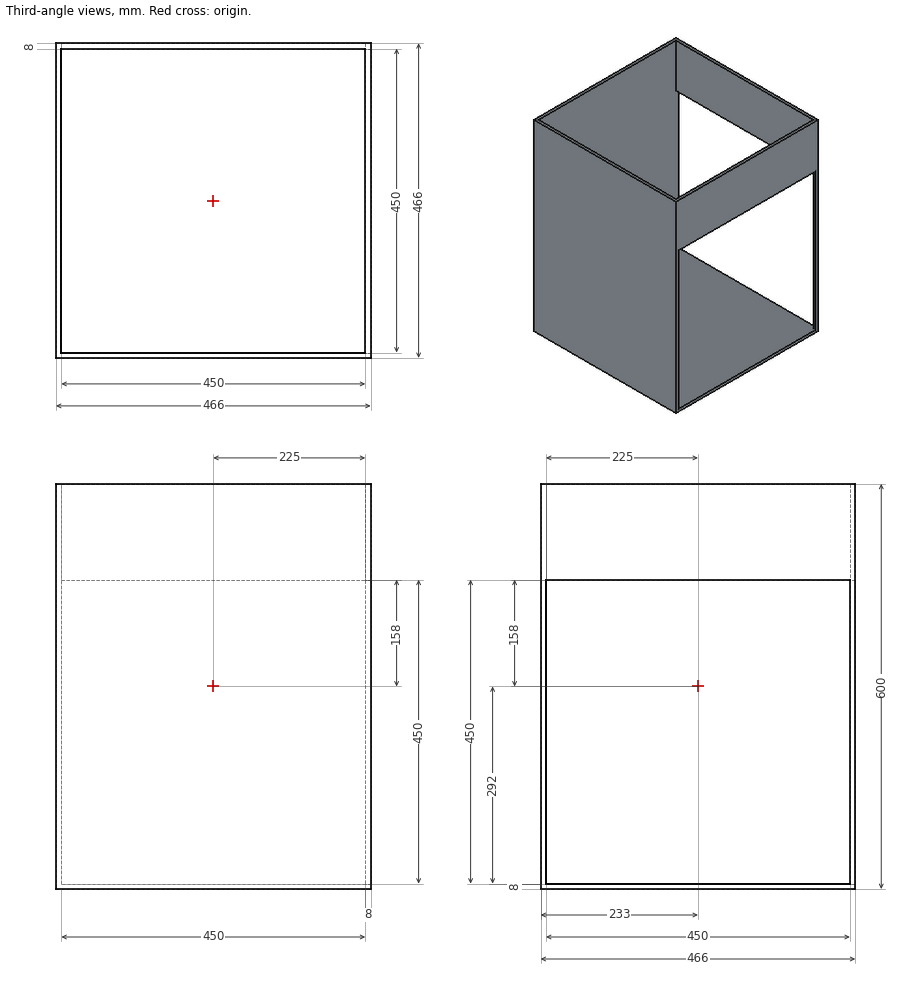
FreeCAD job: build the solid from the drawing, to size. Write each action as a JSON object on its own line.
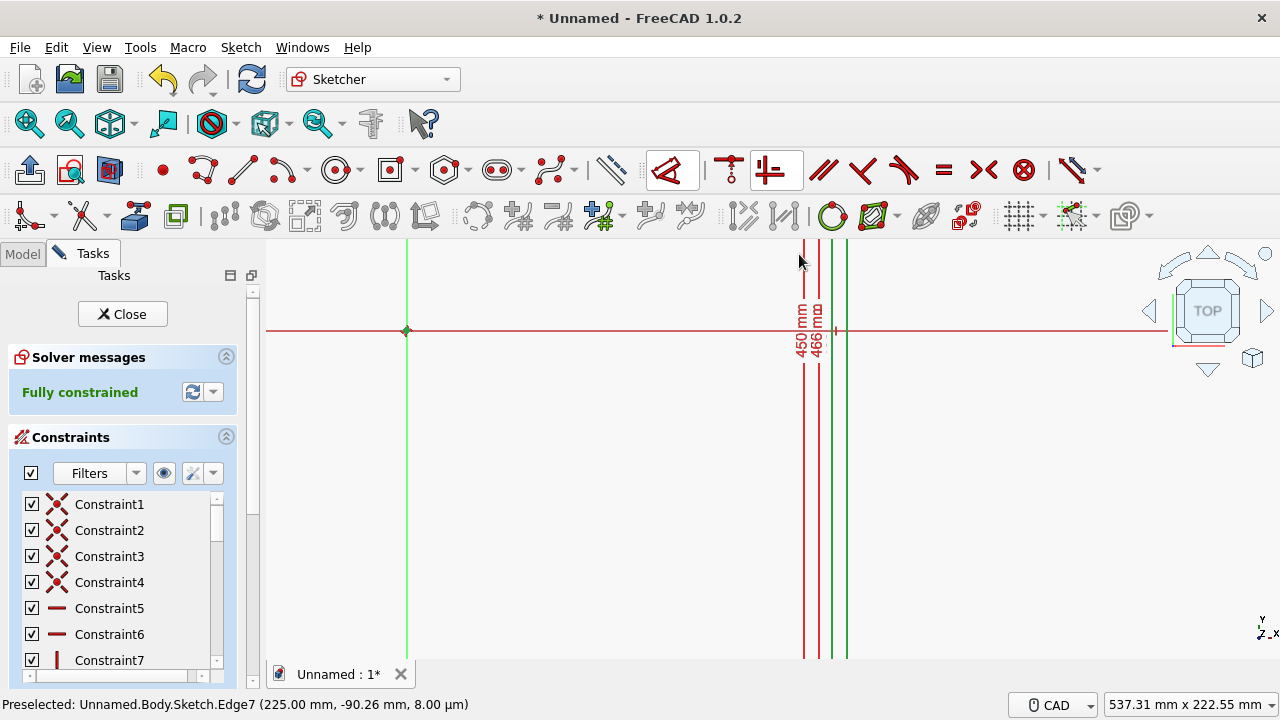
{"action": "left_click", "coordinate": [123, 314]}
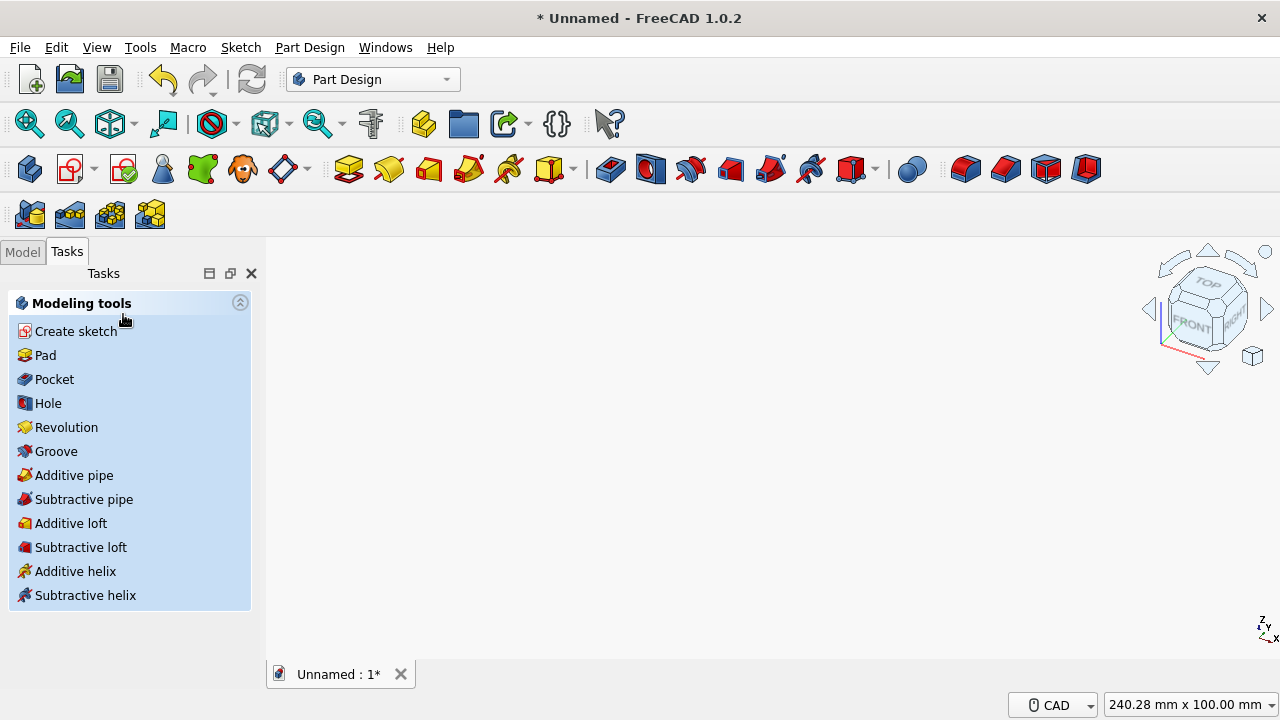
{"action": "left_click", "coordinate": [350, 170]}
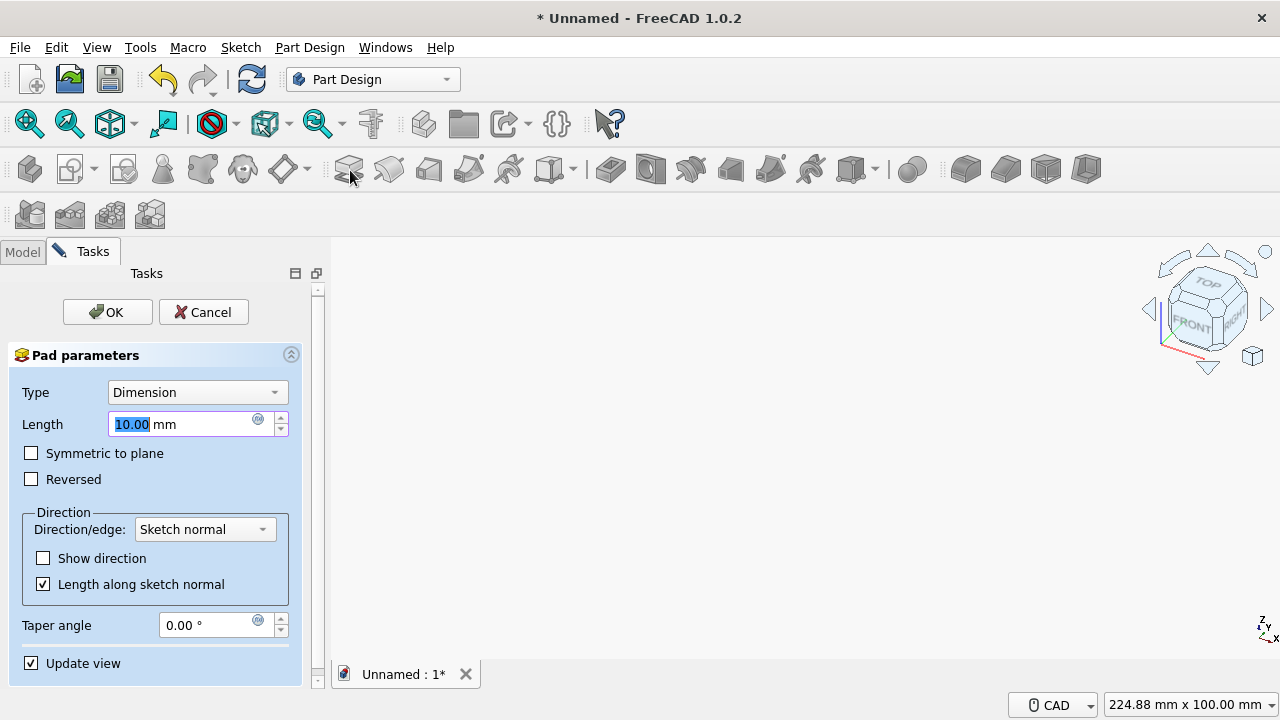
{"action": "type", "text": "600"}
{"action": "key", "text": "Tab"}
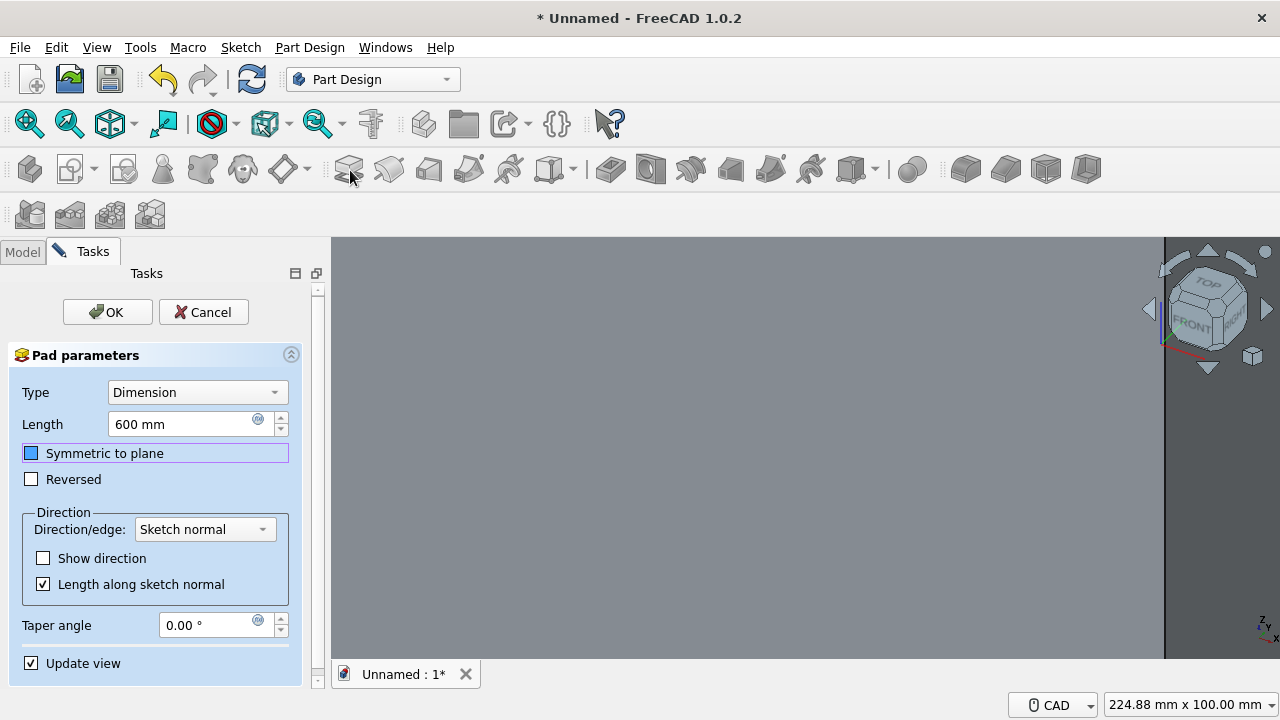
{"action": "left_click", "coordinate": [30, 453]}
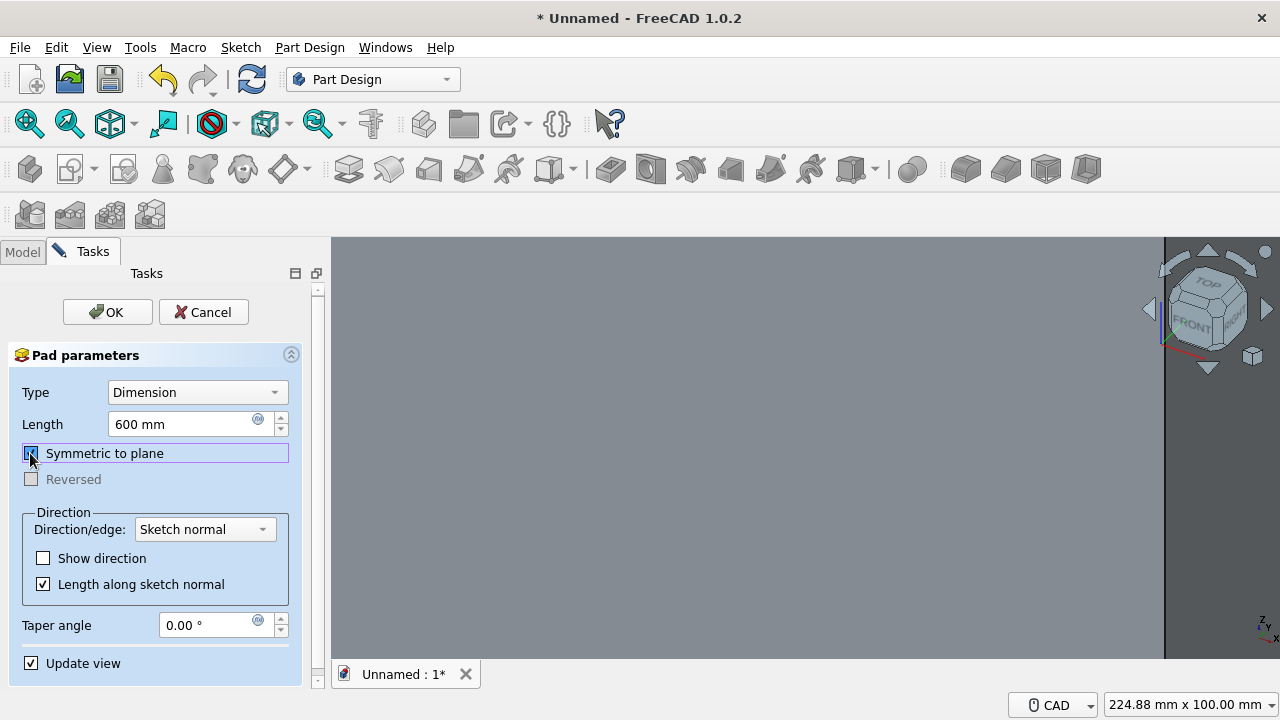
{"action": "left_click", "coordinate": [108, 312]}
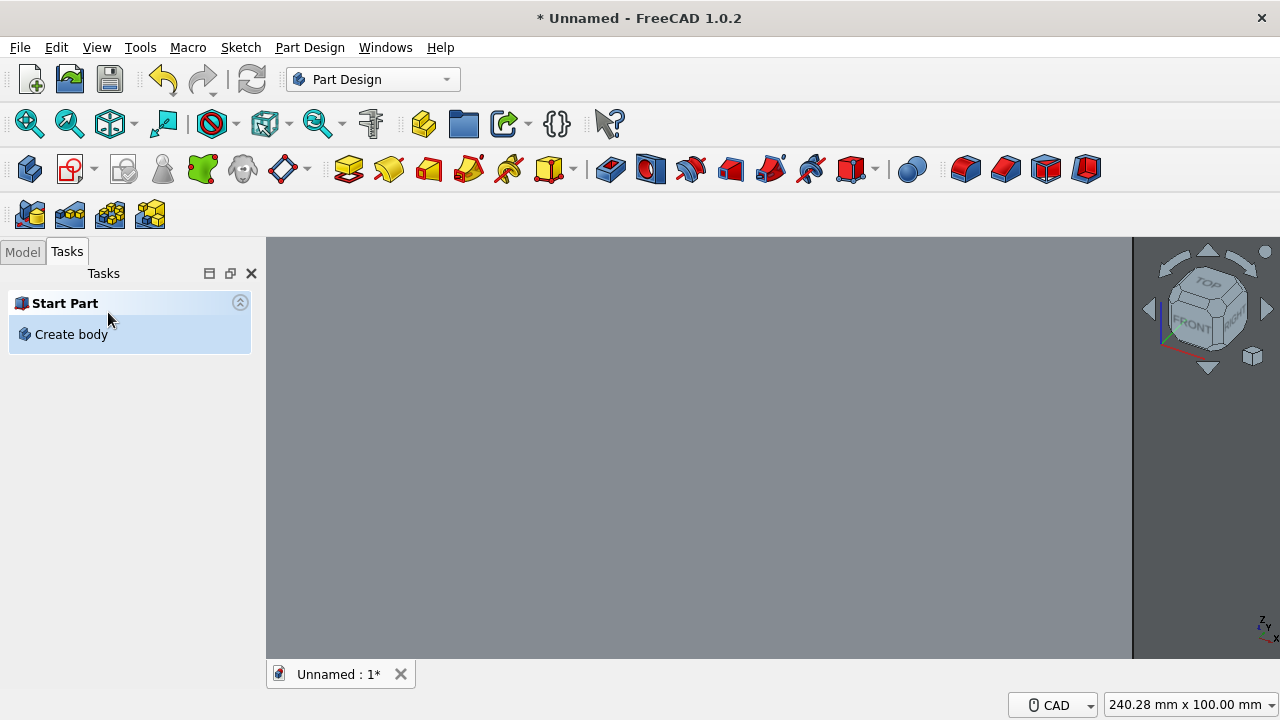
{"action": "left_click", "coordinate": [30, 124]}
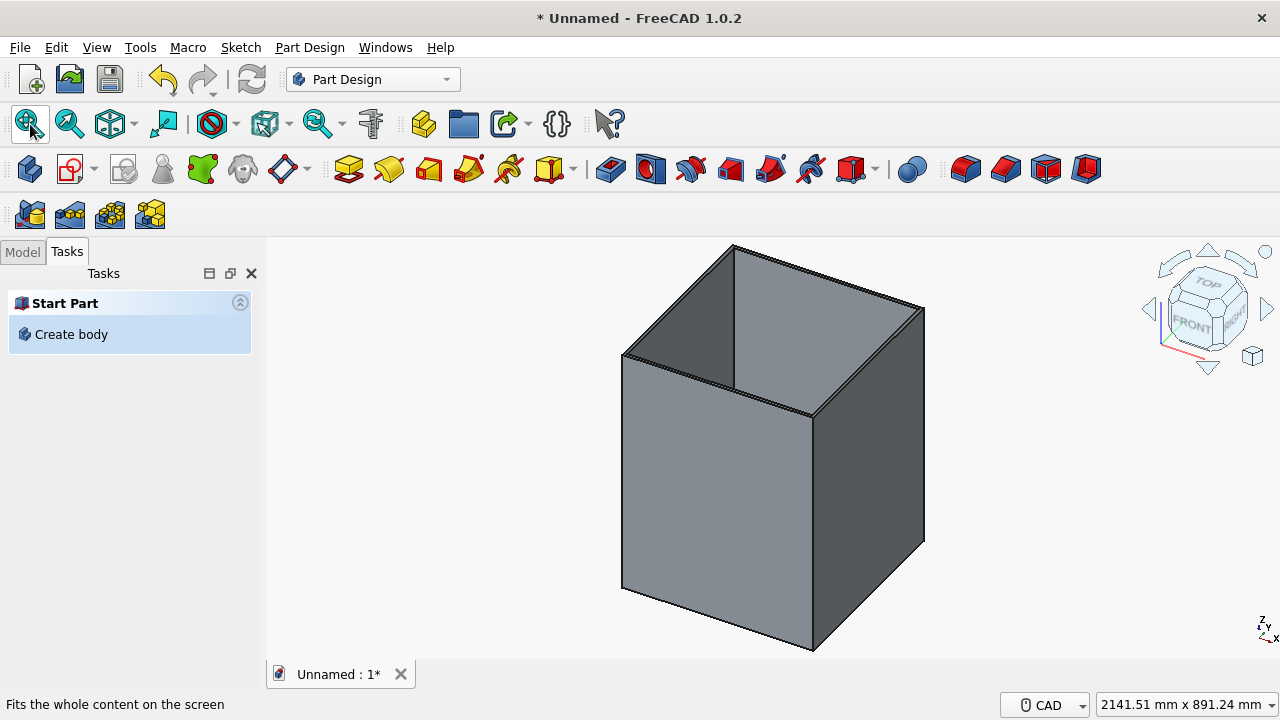
{"action": "left_click", "coordinate": [23, 251]}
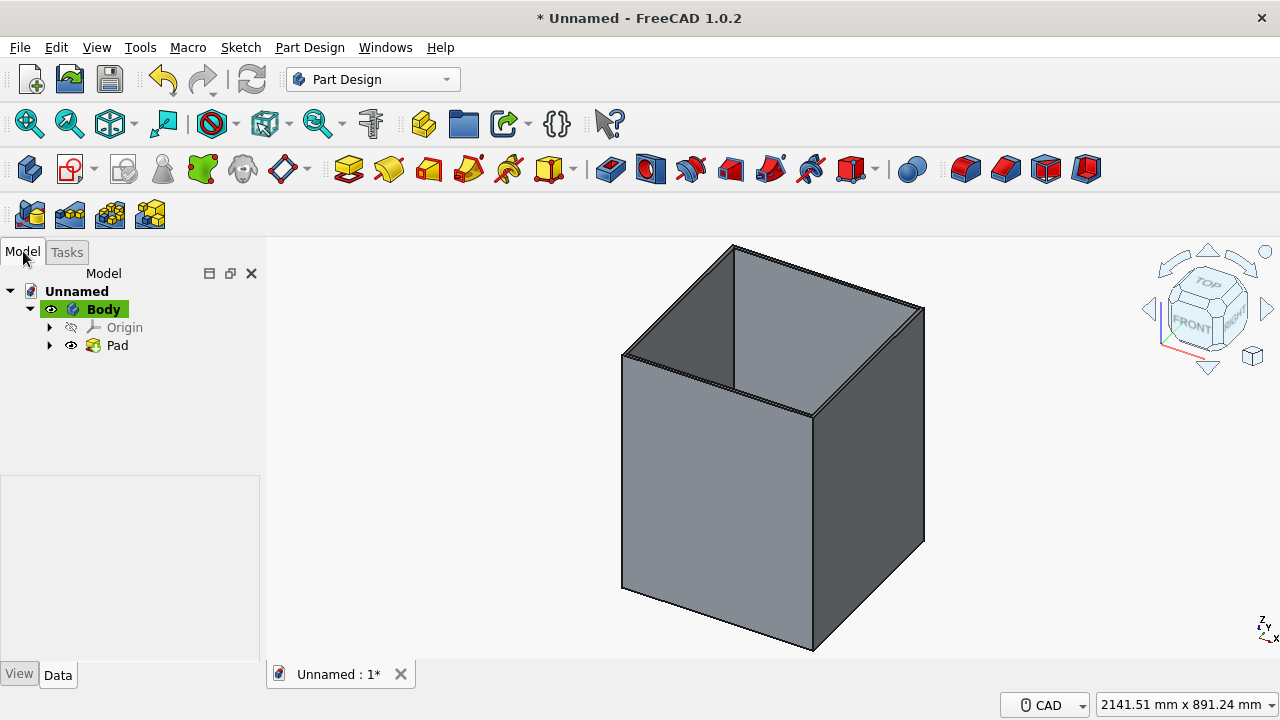
{"action": "left_click", "coordinate": [50, 327]}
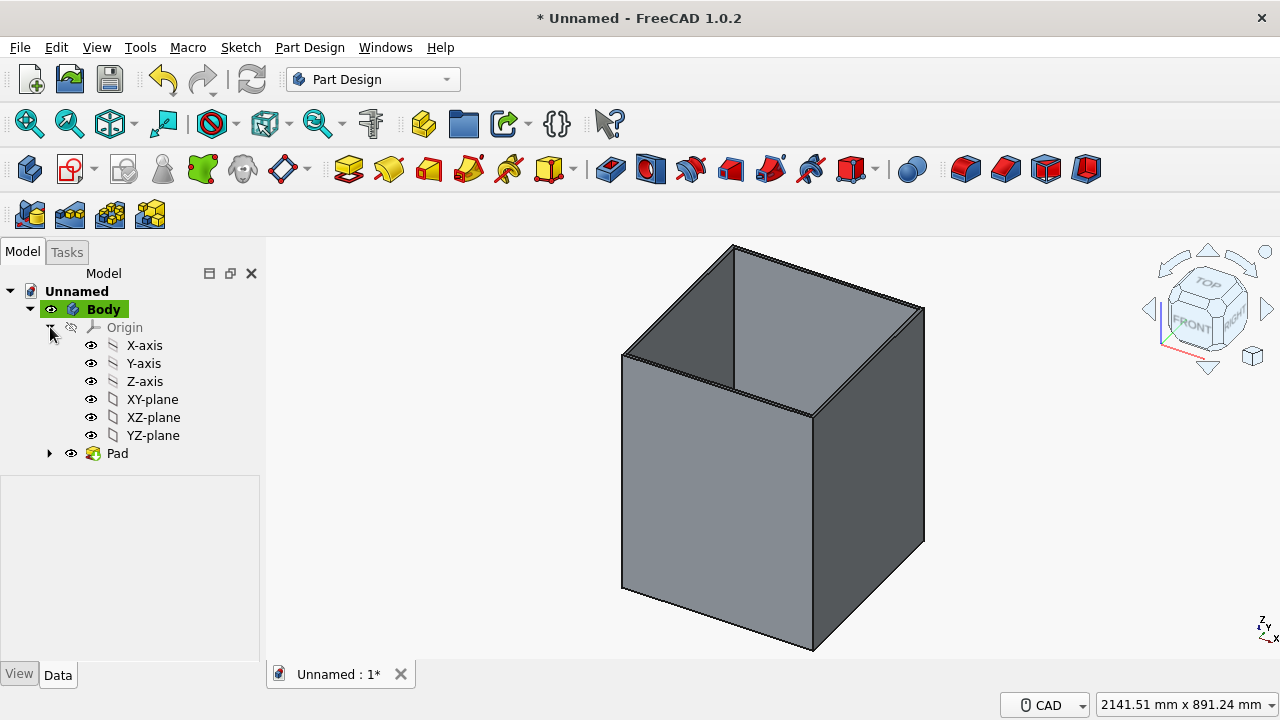
{"action": "left_click", "coordinate": [136, 435]}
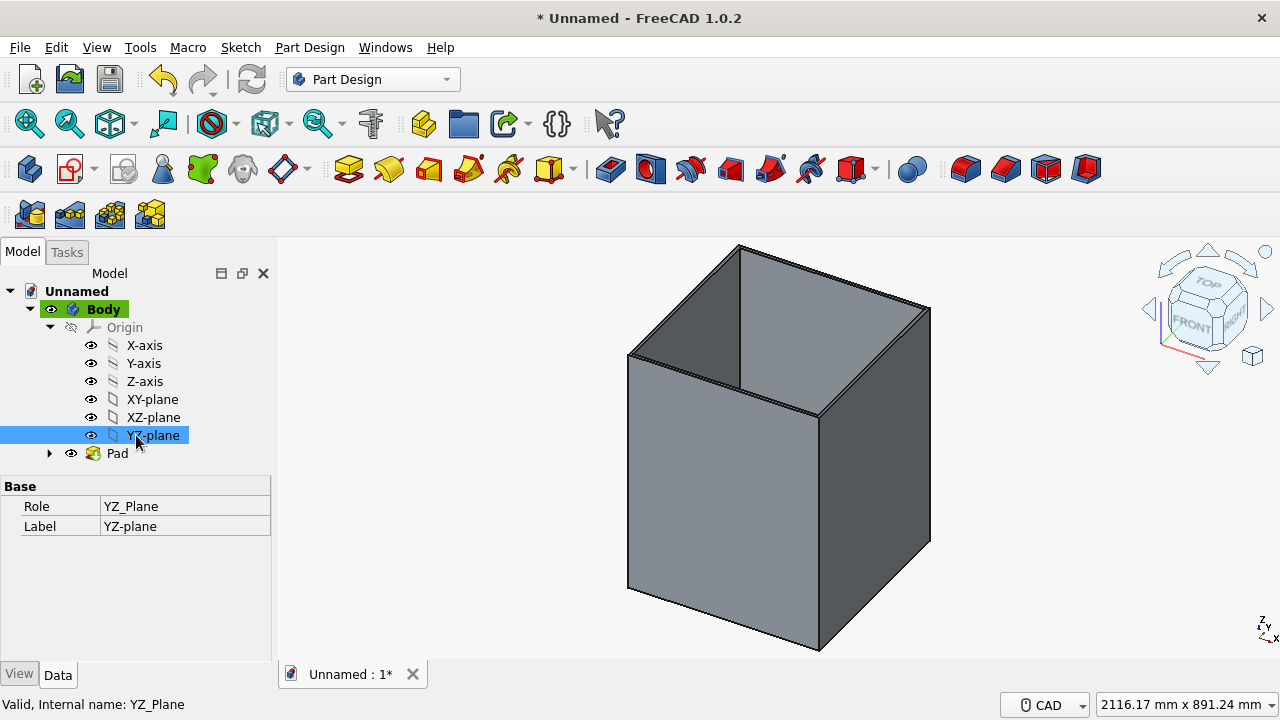
{"action": "left_click", "coordinate": [284, 170]}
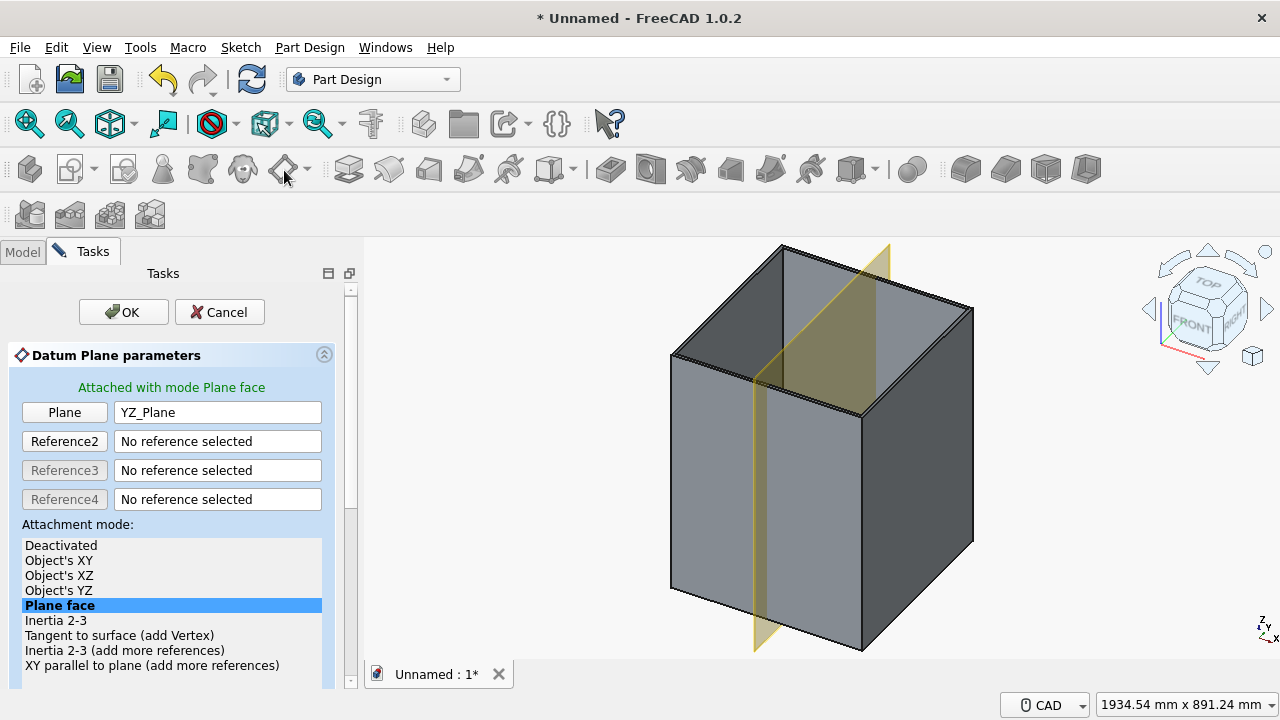
{"action": "scroll", "coordinate": [351, 486], "scroll_direction": "down", "scroll_amount": 4}